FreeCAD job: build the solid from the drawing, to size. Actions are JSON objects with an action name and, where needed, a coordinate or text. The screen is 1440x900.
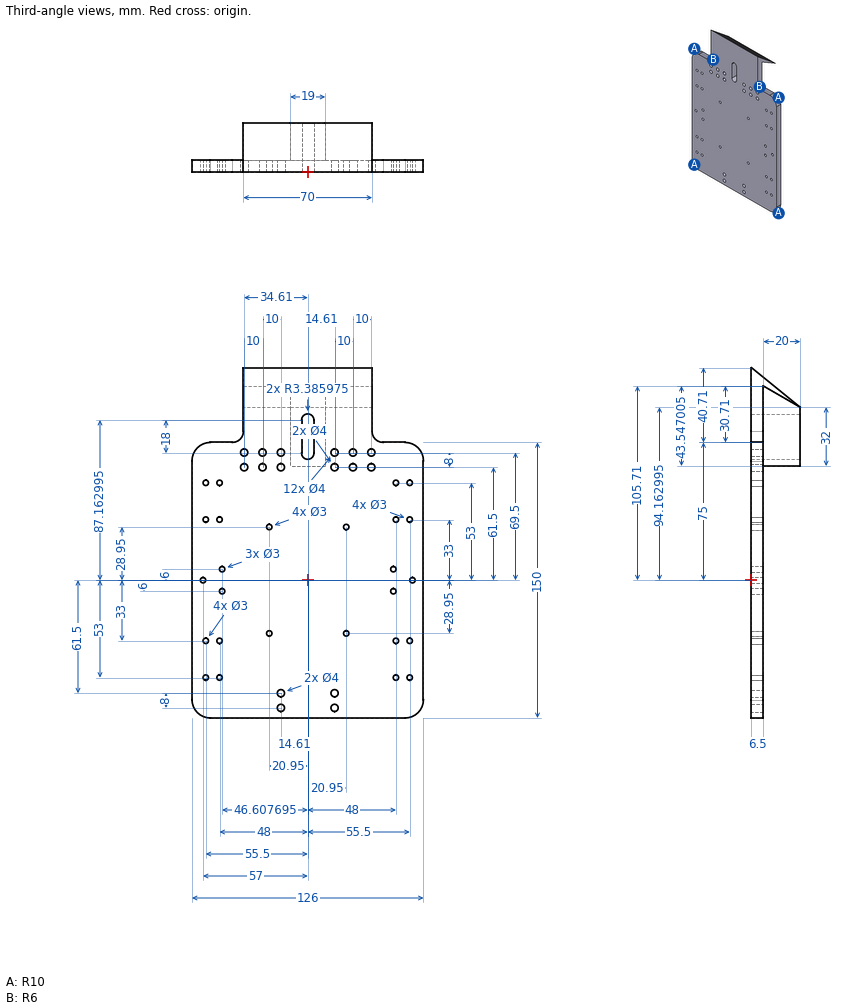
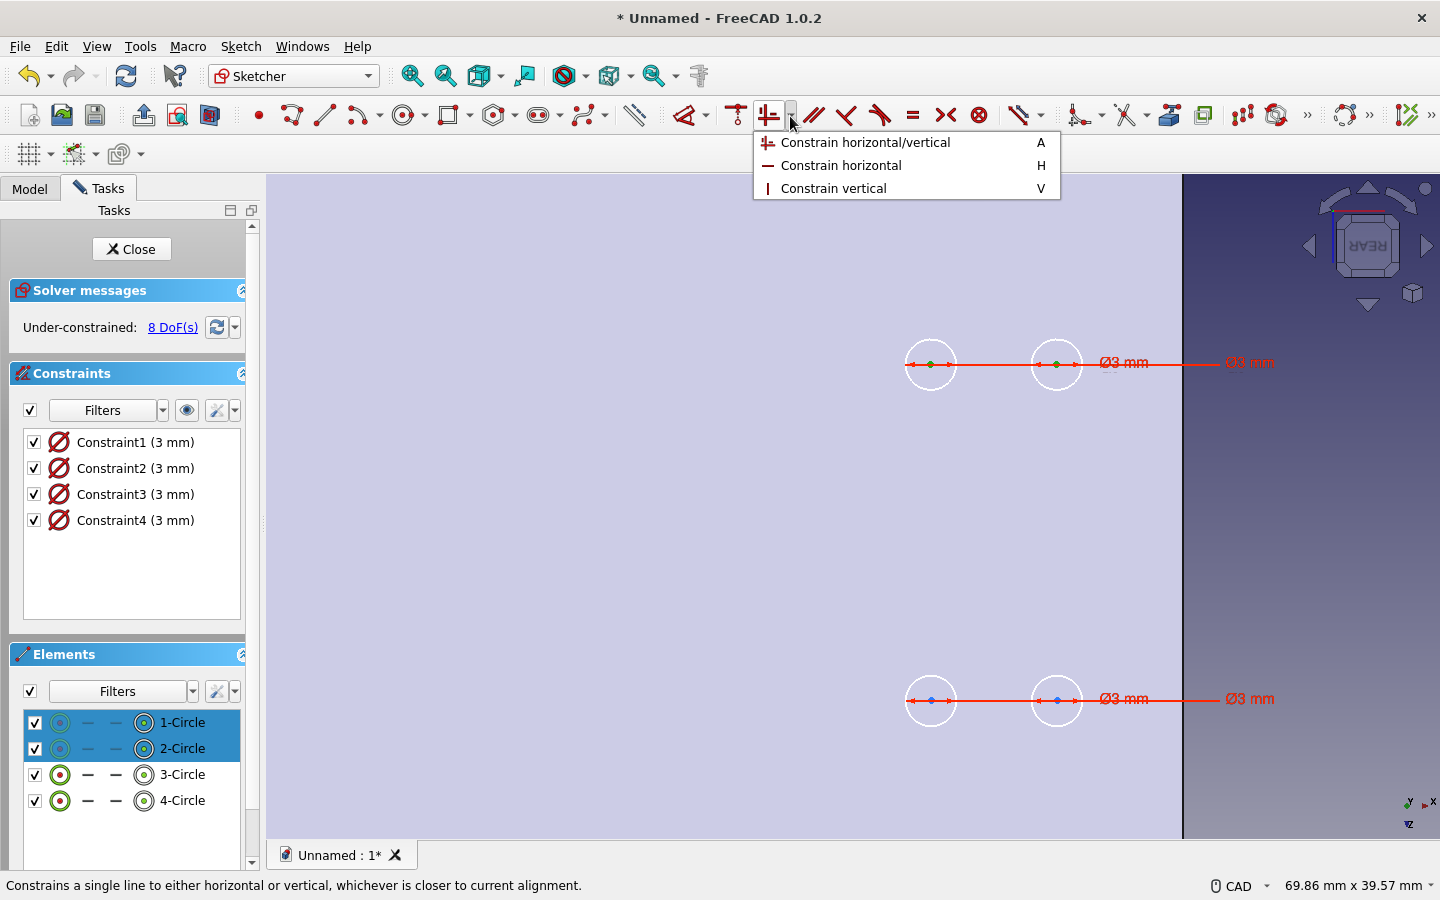
{"action": "left_click", "coordinate": [907, 166]}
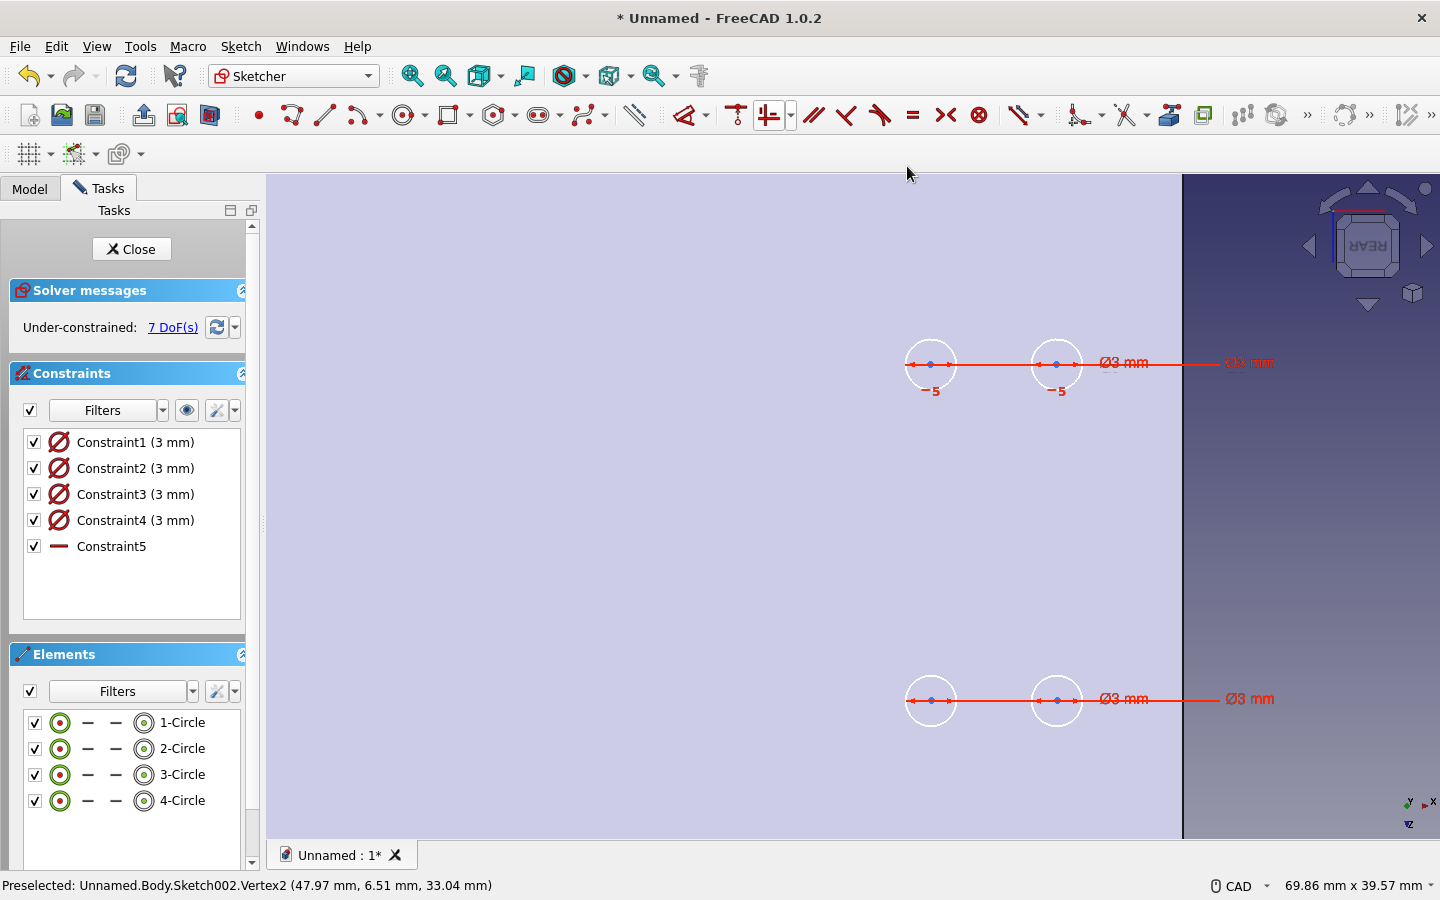
{"action": "left_click", "coordinate": [931, 365]}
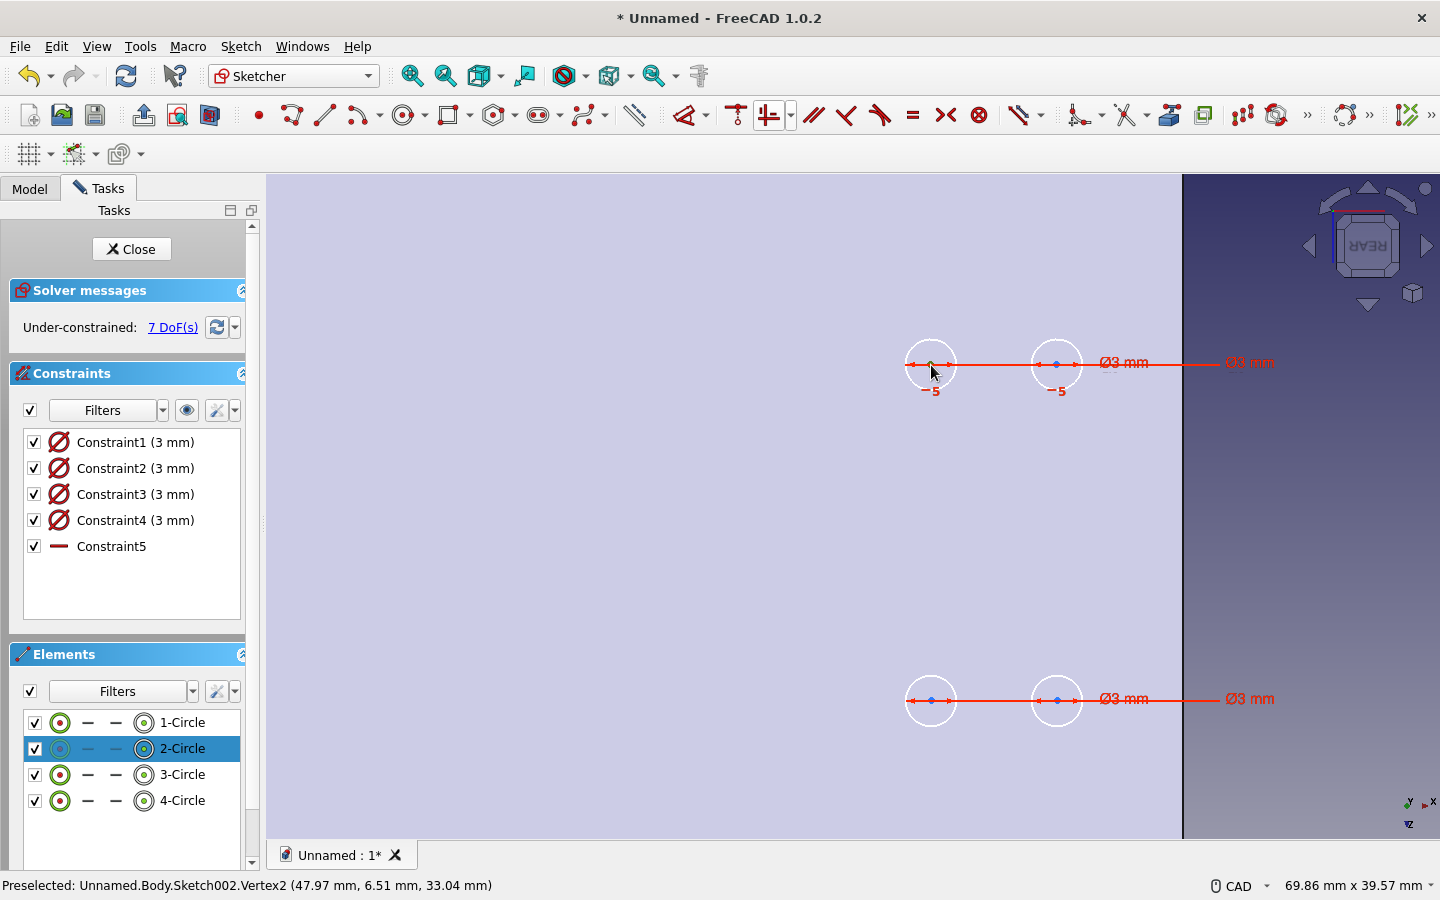
{"action": "left_click", "coordinate": [931, 701]}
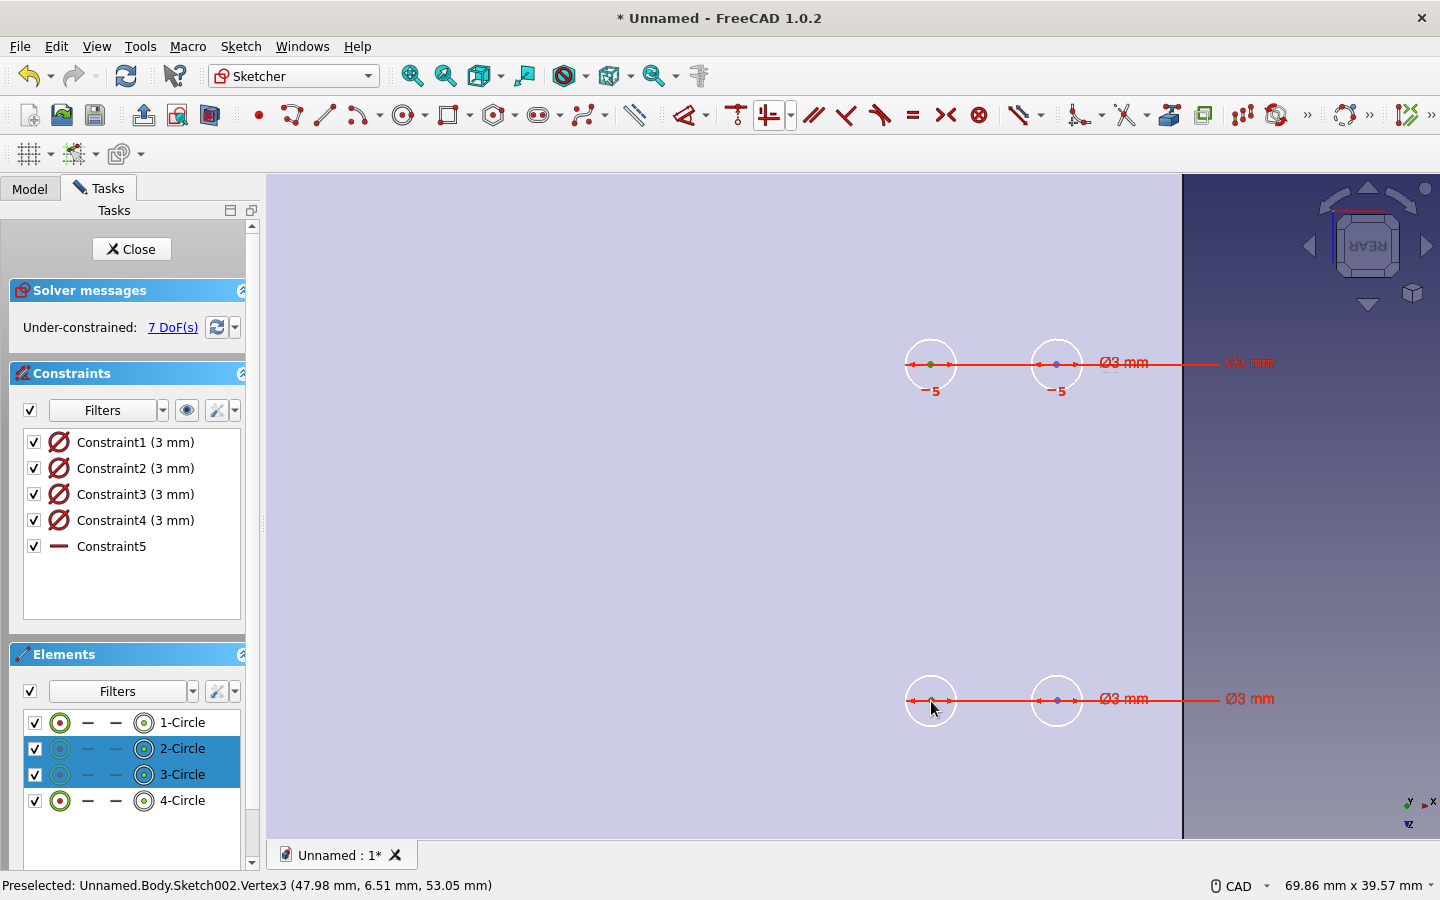
{"action": "left_click", "coordinate": [790, 116]}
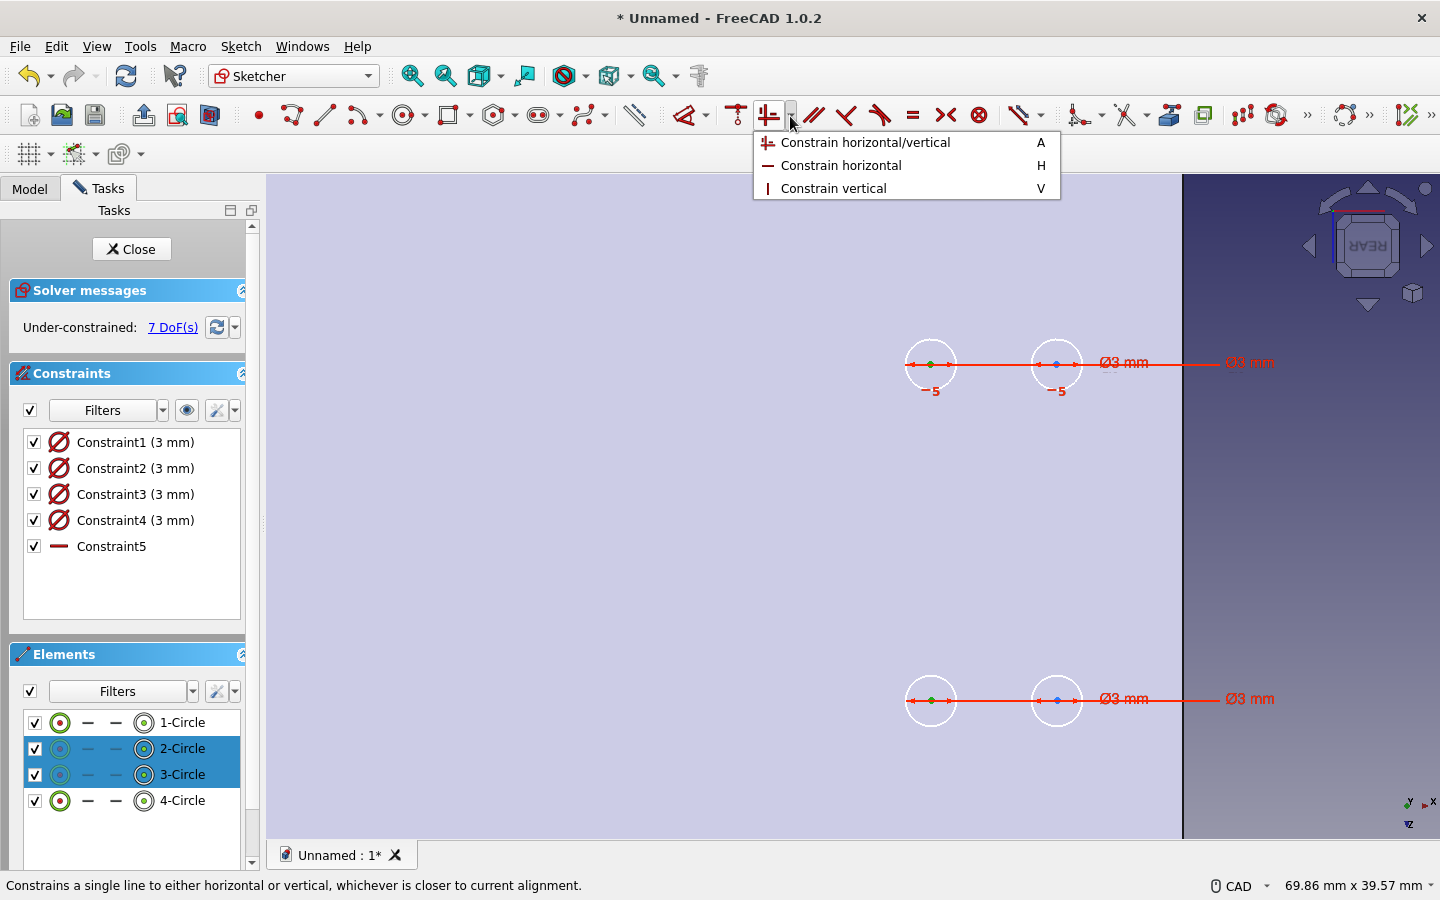
{"action": "left_click", "coordinate": [907, 188]}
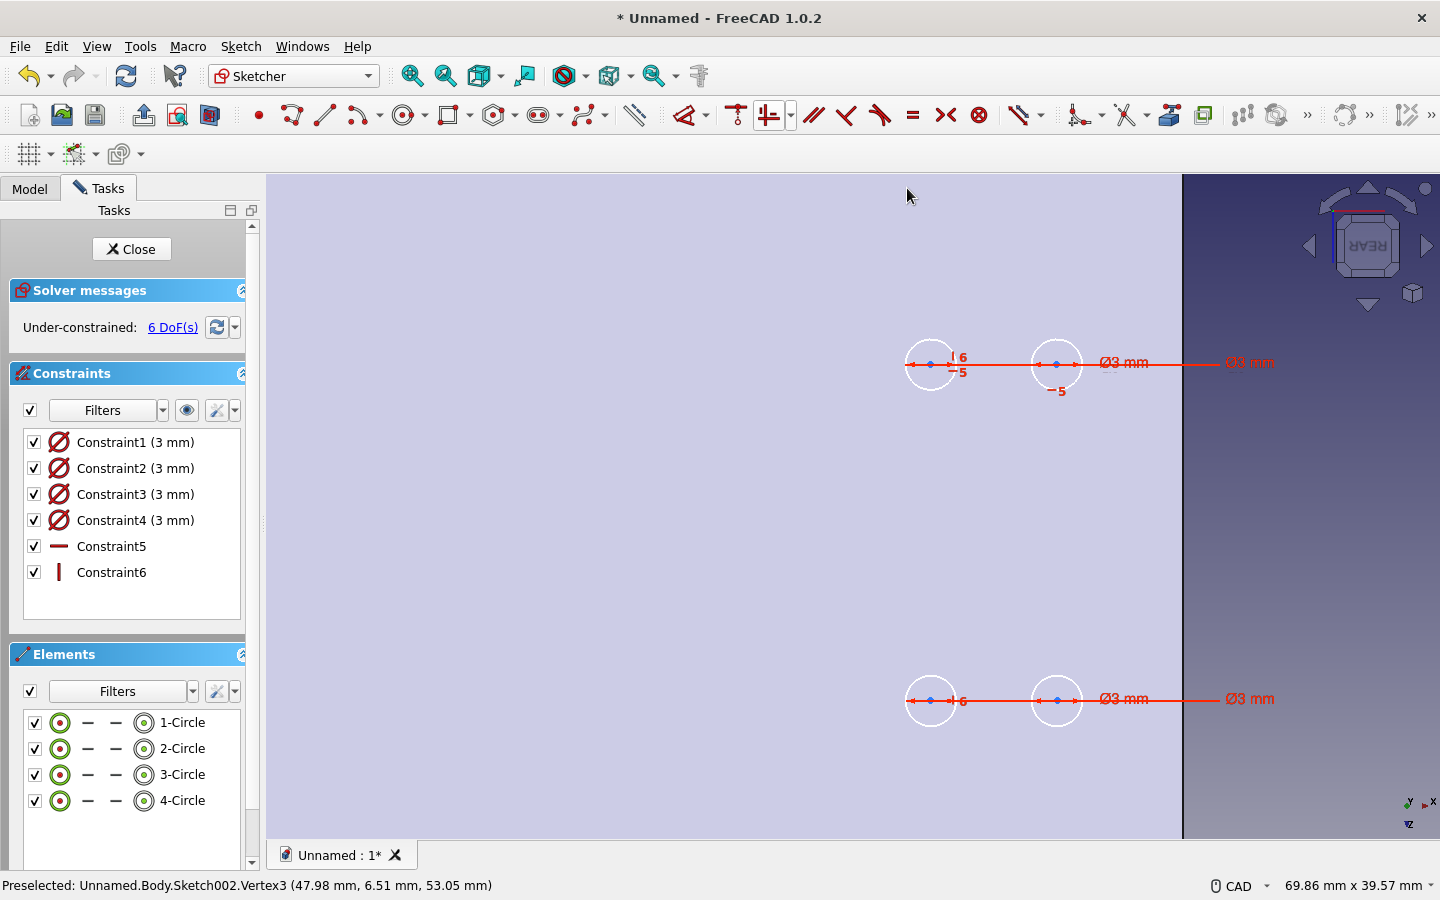
{"action": "left_click", "coordinate": [1057, 365]}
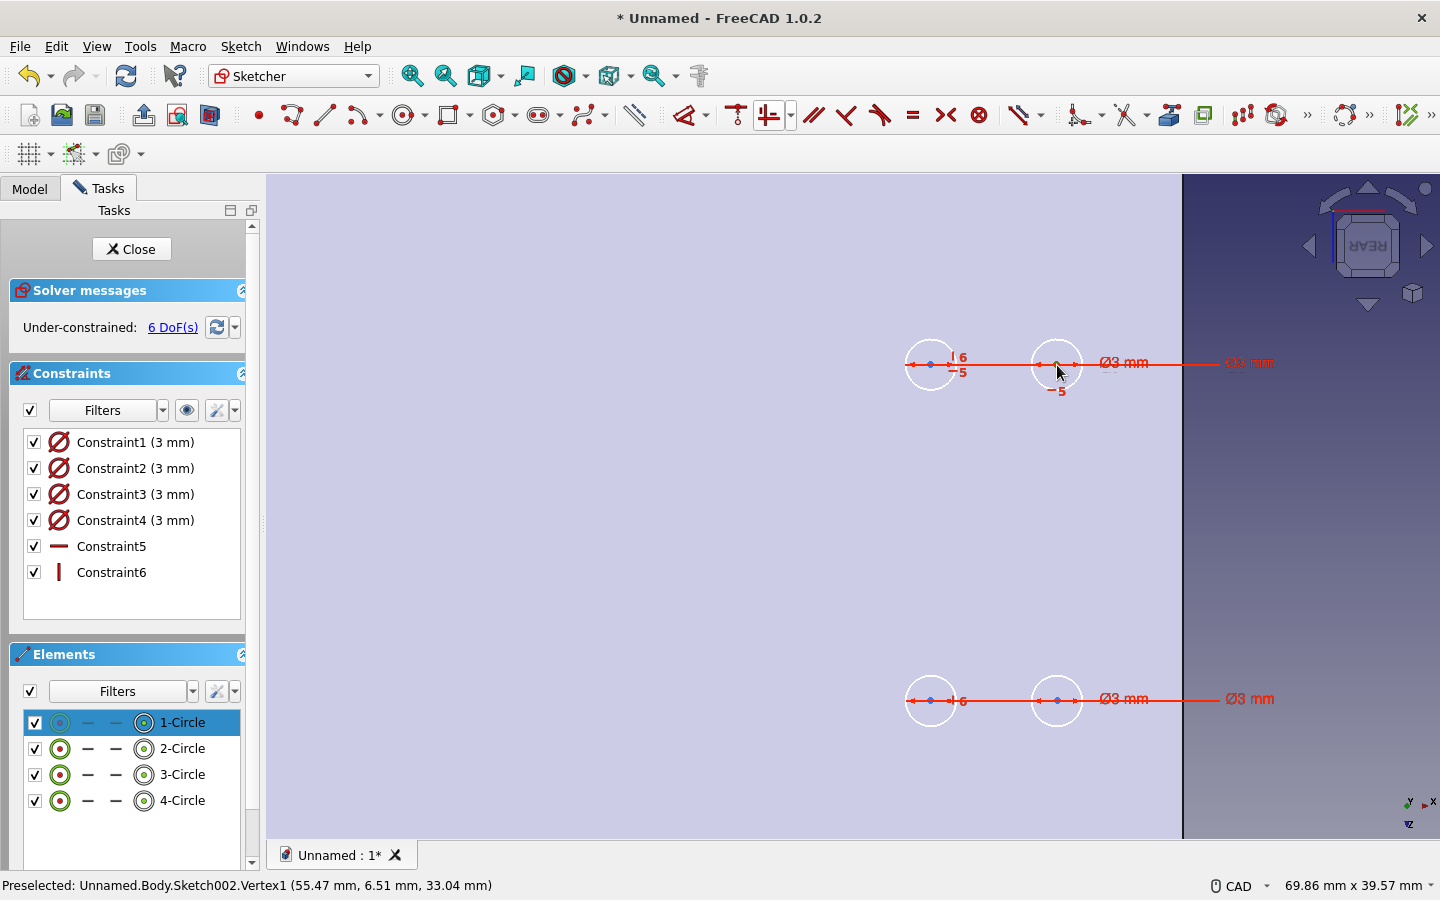
{"action": "left_click", "coordinate": [1057, 701]}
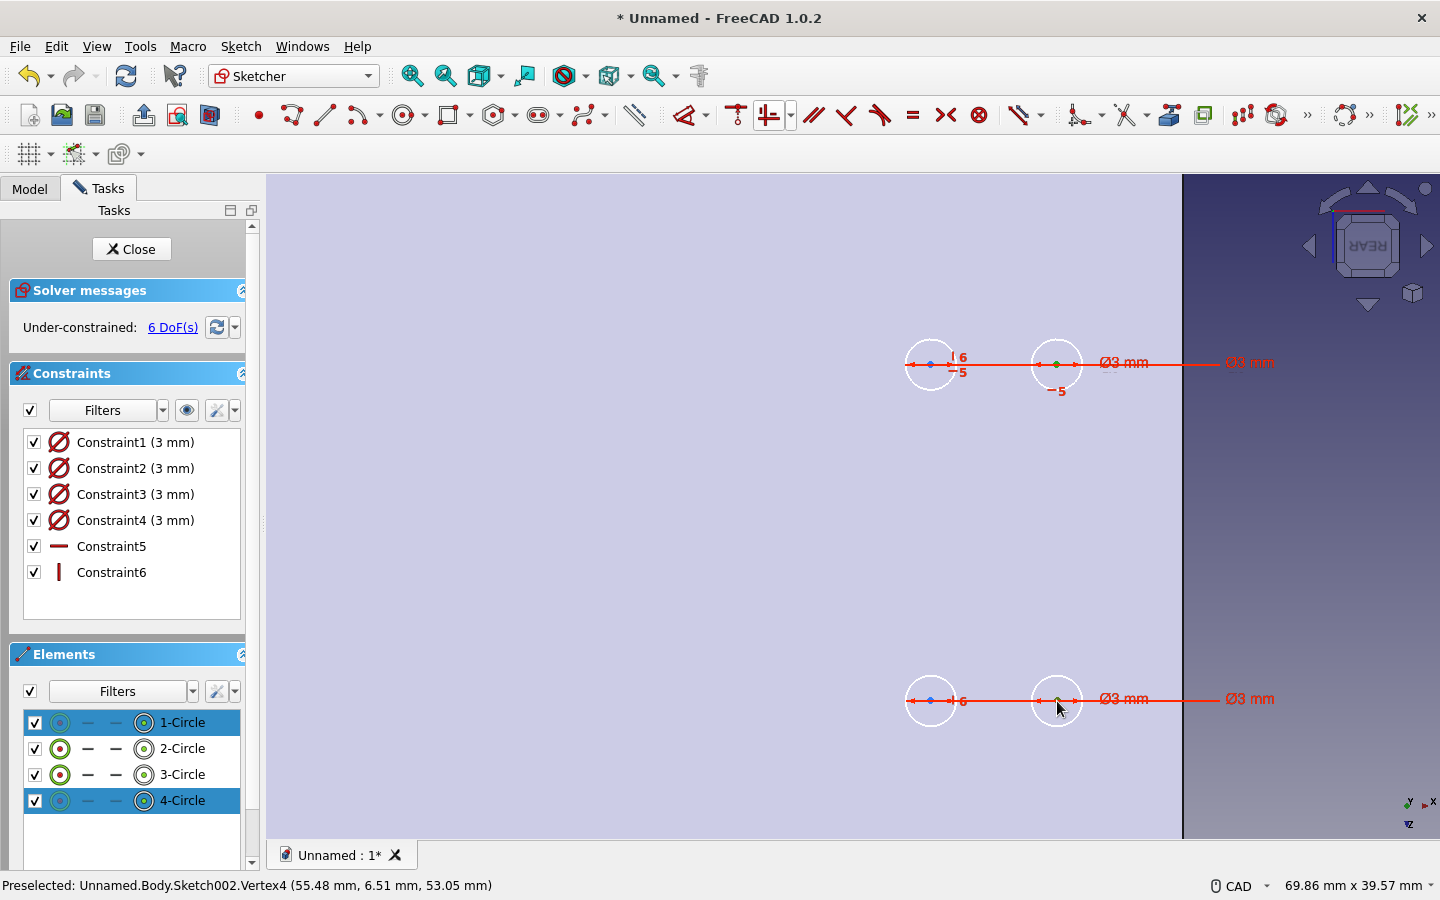
{"action": "left_click", "coordinate": [790, 116]}